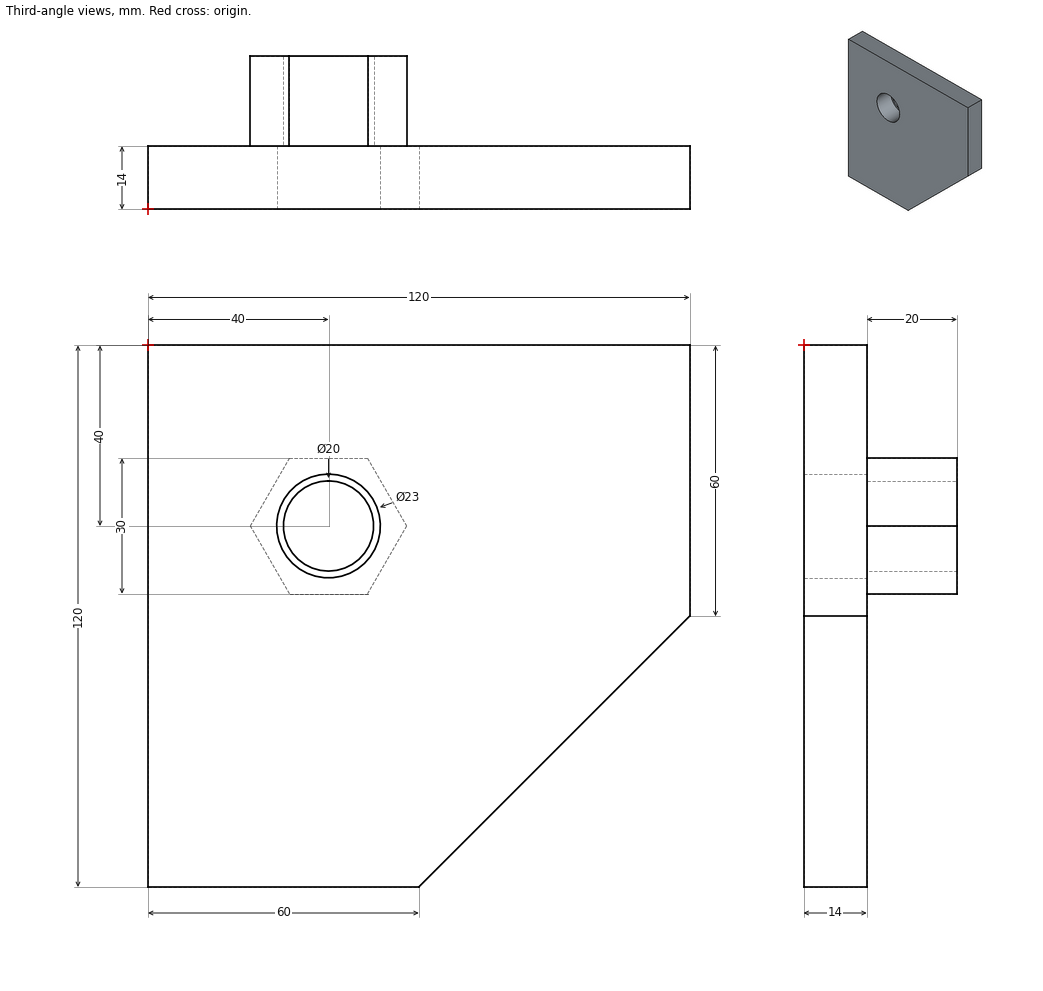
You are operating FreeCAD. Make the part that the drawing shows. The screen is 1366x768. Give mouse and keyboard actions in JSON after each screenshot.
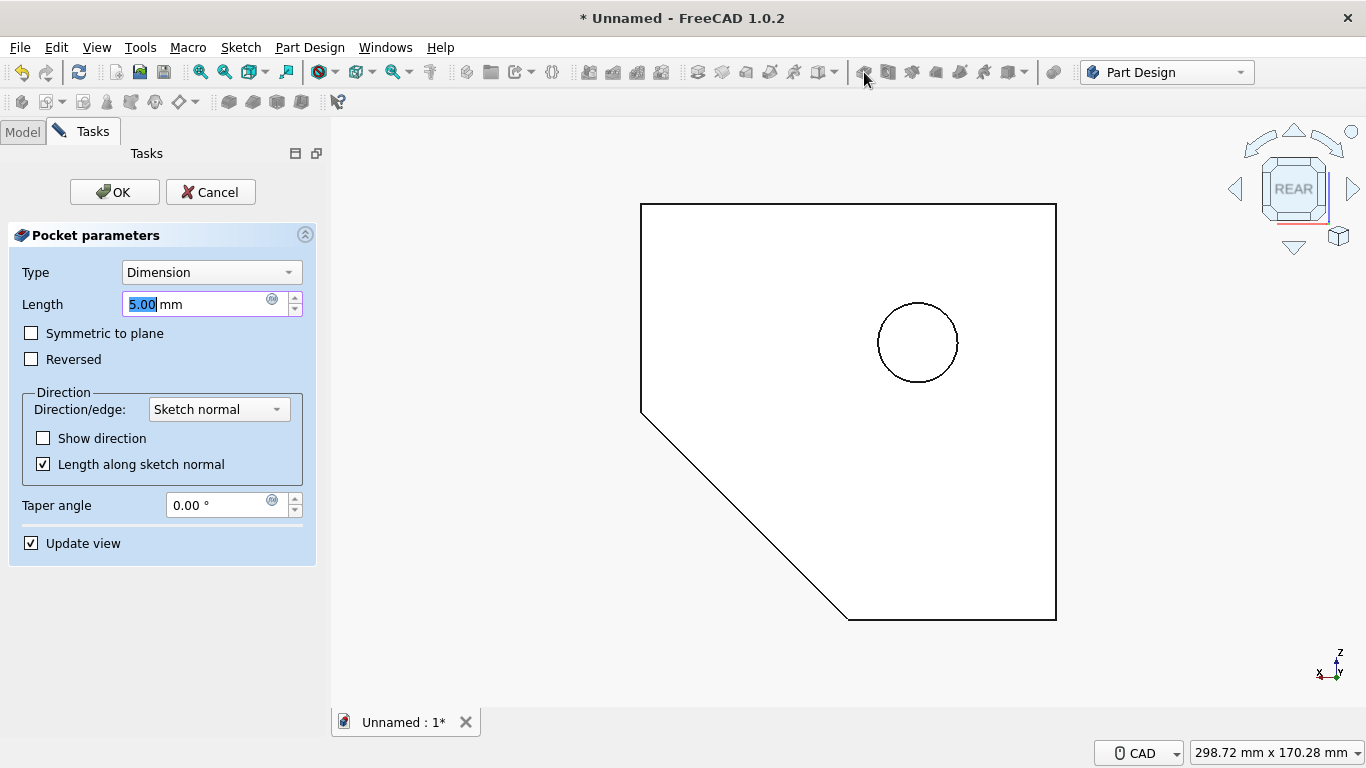
{"action": "type", "text": "14"}
{"action": "key", "text": "Tab"}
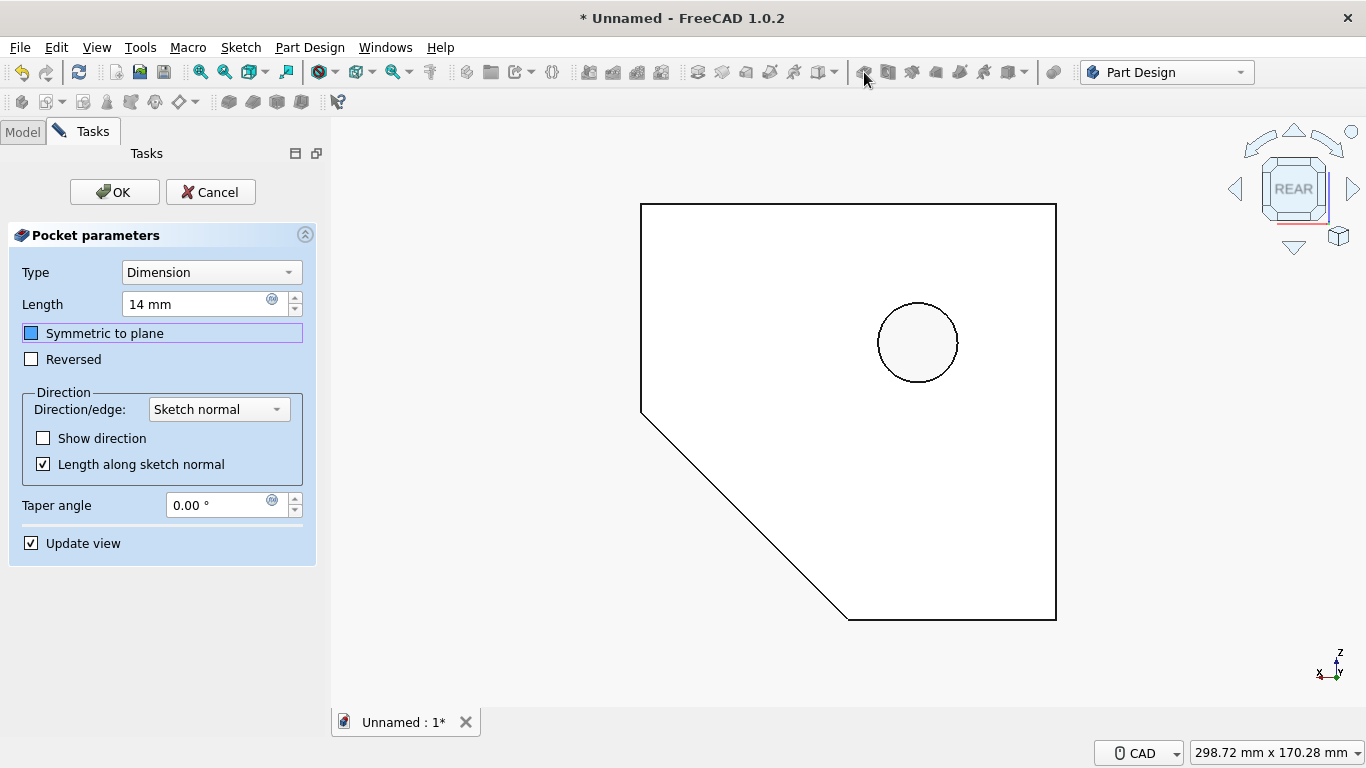
{"action": "left_click", "coordinate": [115, 192]}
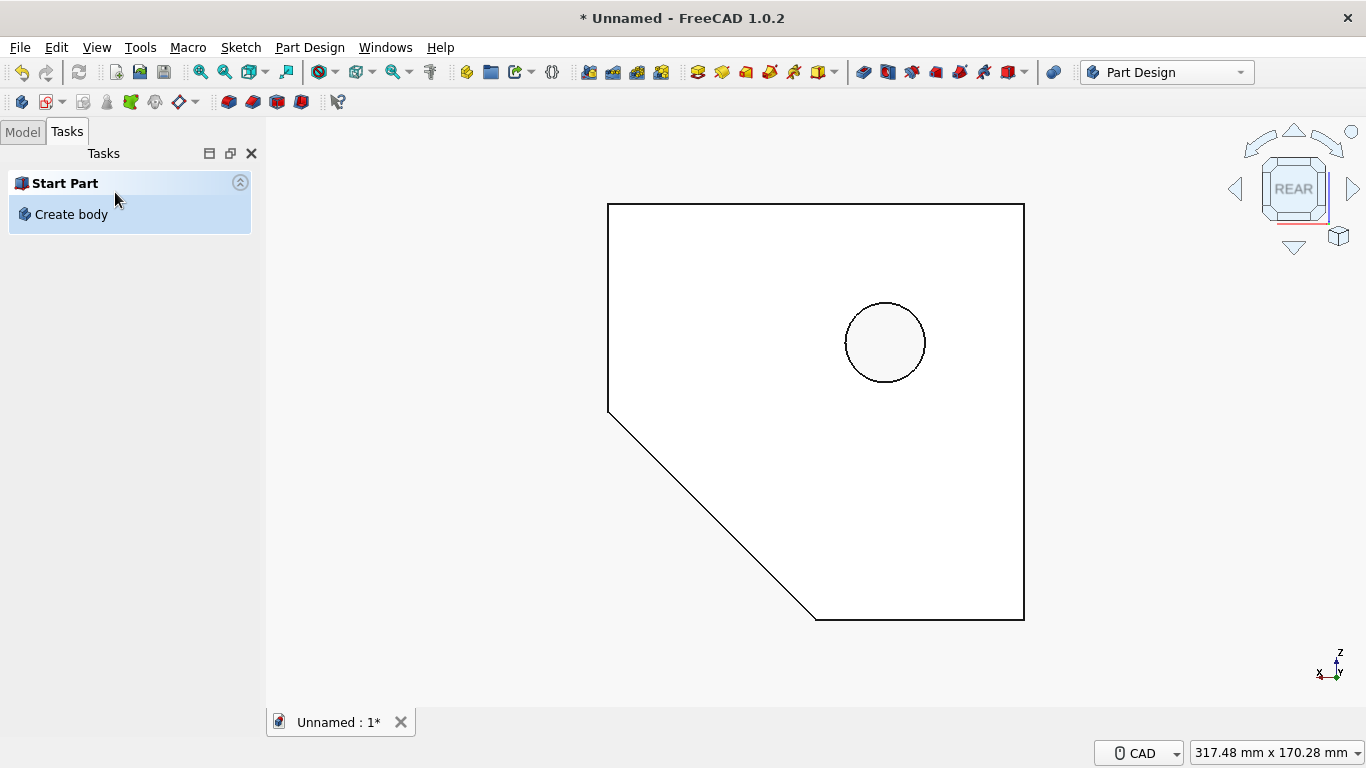
{"action": "left_click", "coordinate": [757, 411]}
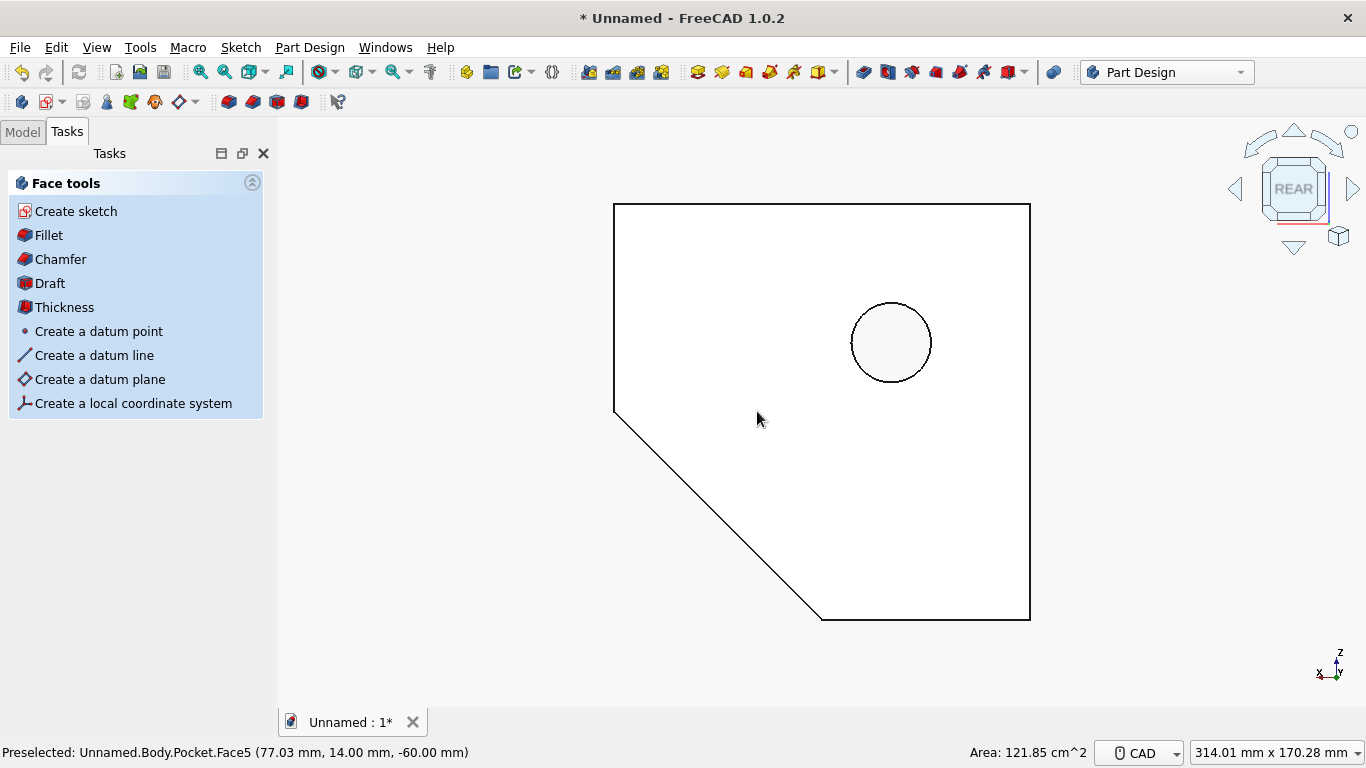
{"action": "left_click", "coordinate": [46, 102]}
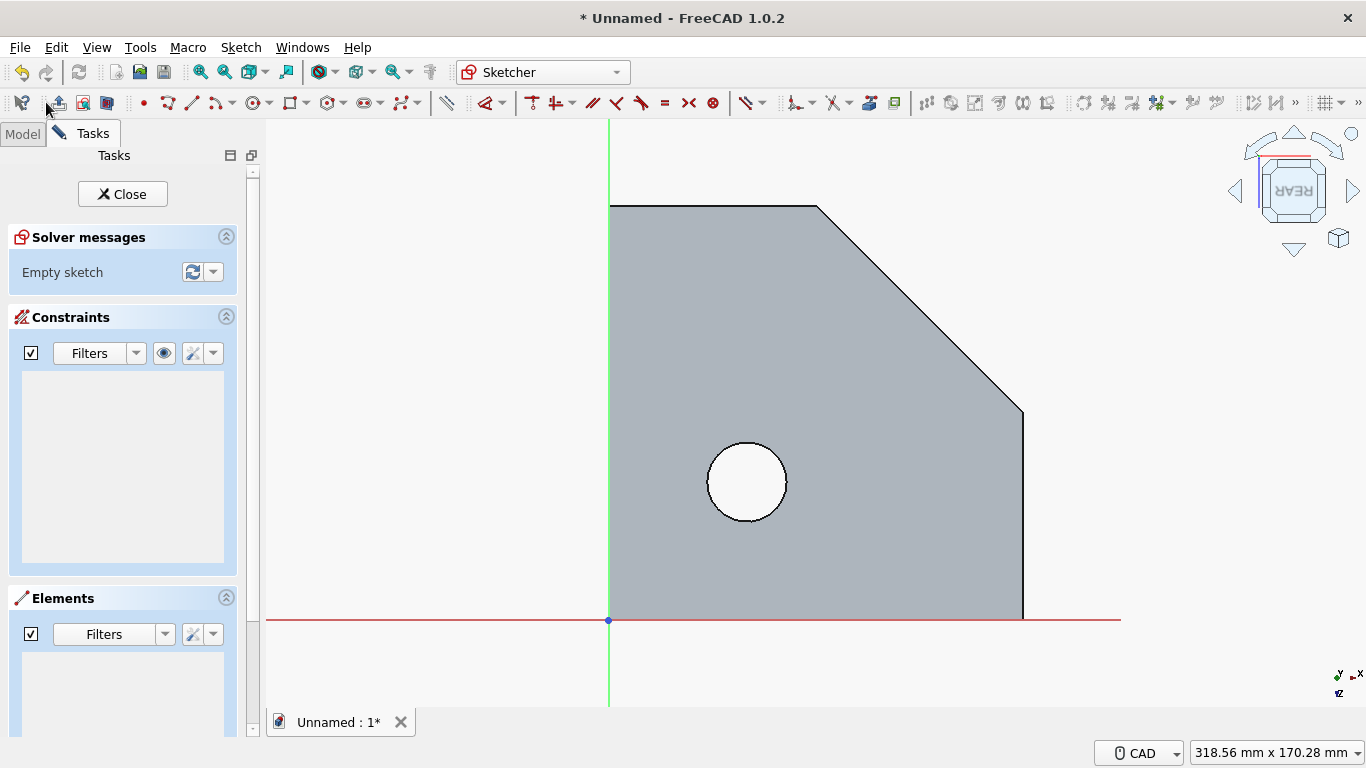
{"action": "scroll", "coordinate": [659, 662], "scroll_direction": "up", "scroll_amount": 3}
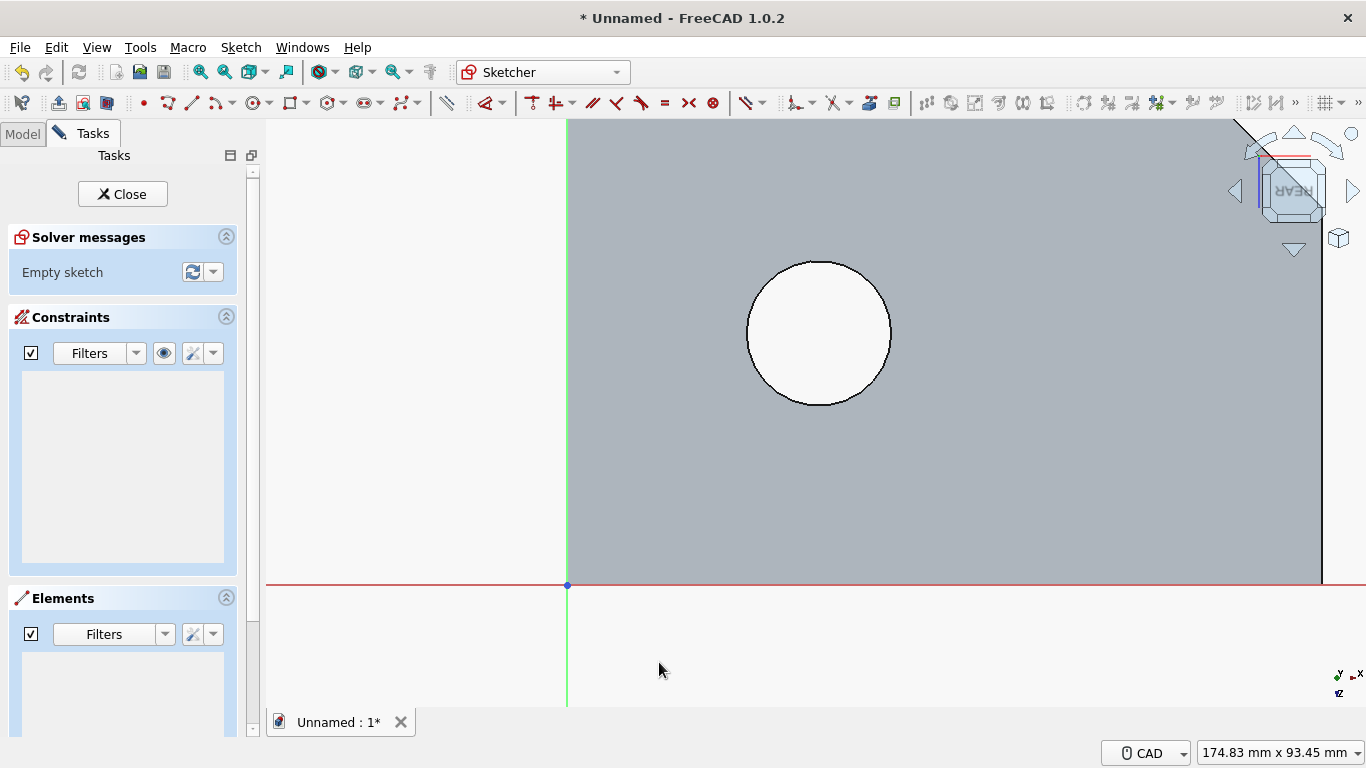
{"action": "left_click", "coordinate": [328, 104]}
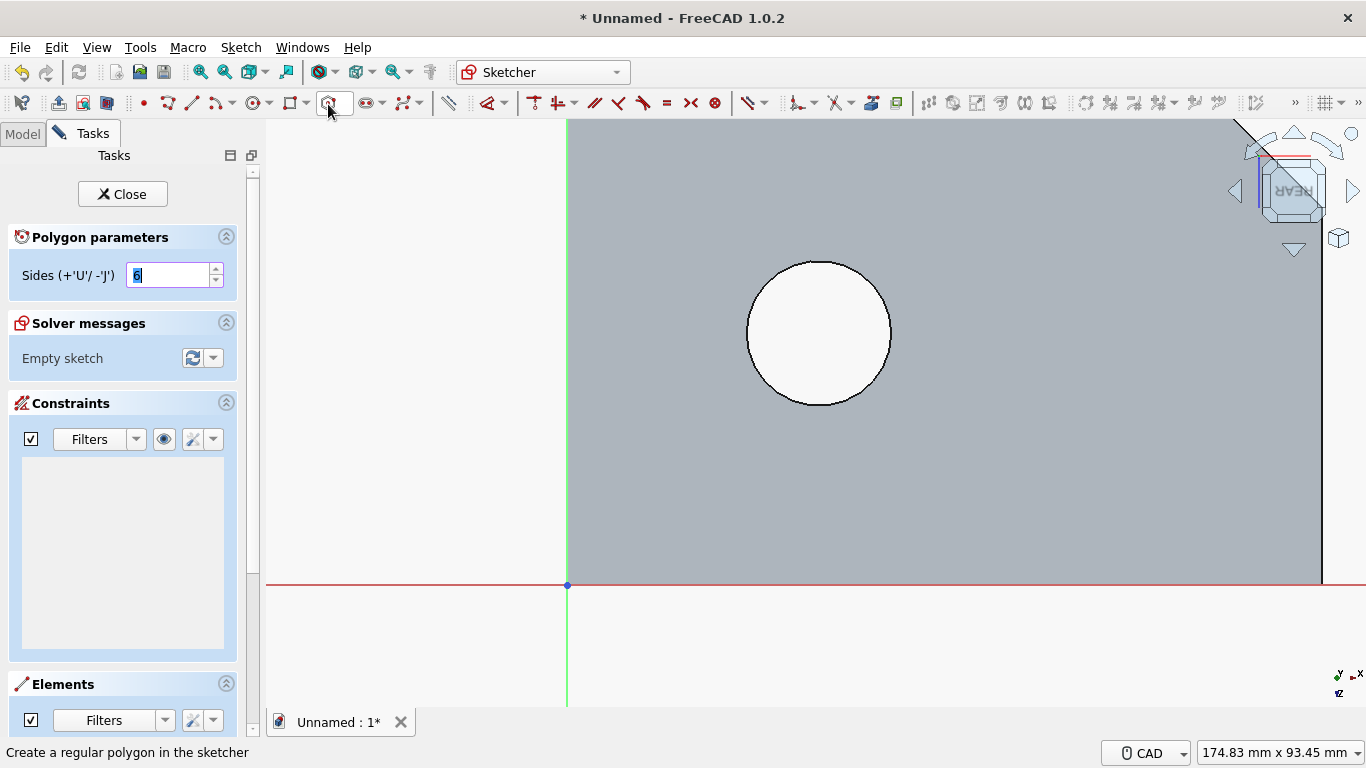
{"action": "left_click", "coordinate": [819, 333]}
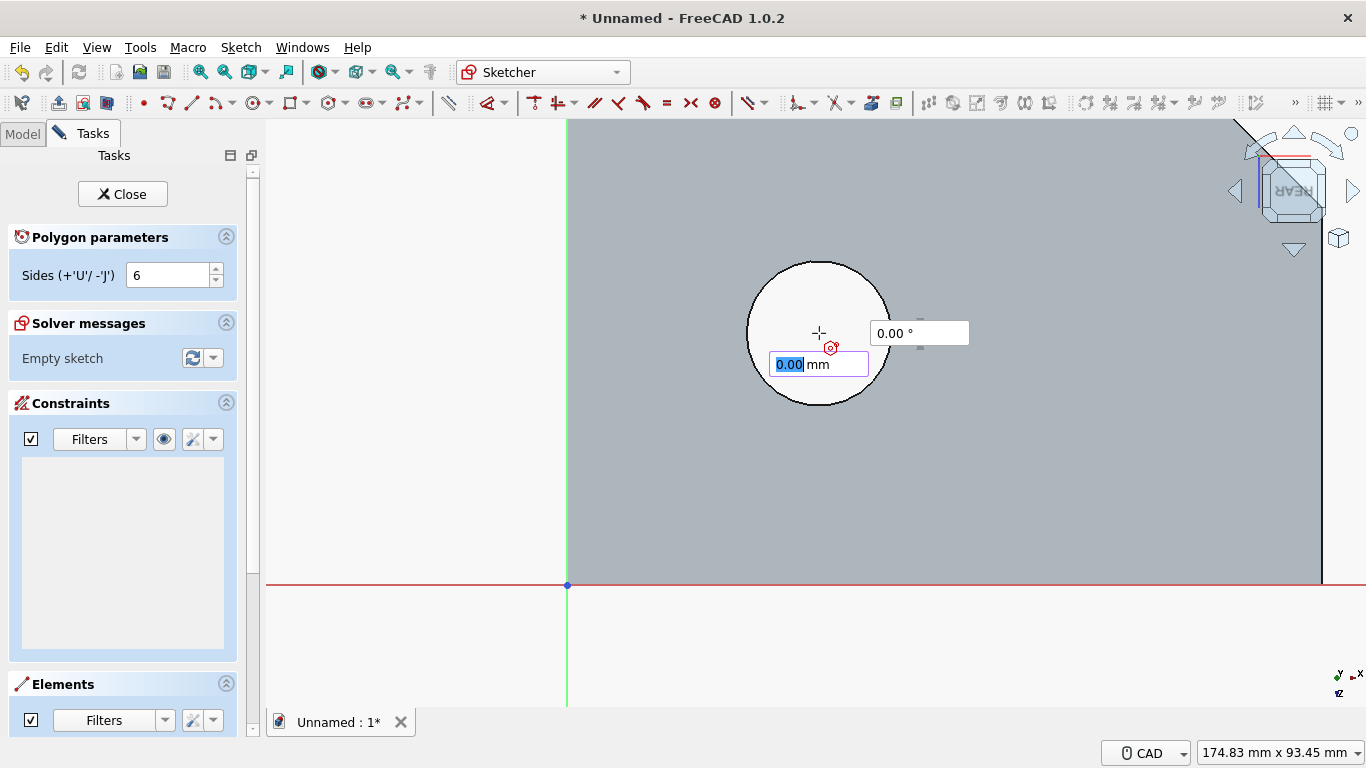
{"action": "left_click", "coordinate": [928, 333]}
{"action": "right_click", "coordinate": [928, 333]}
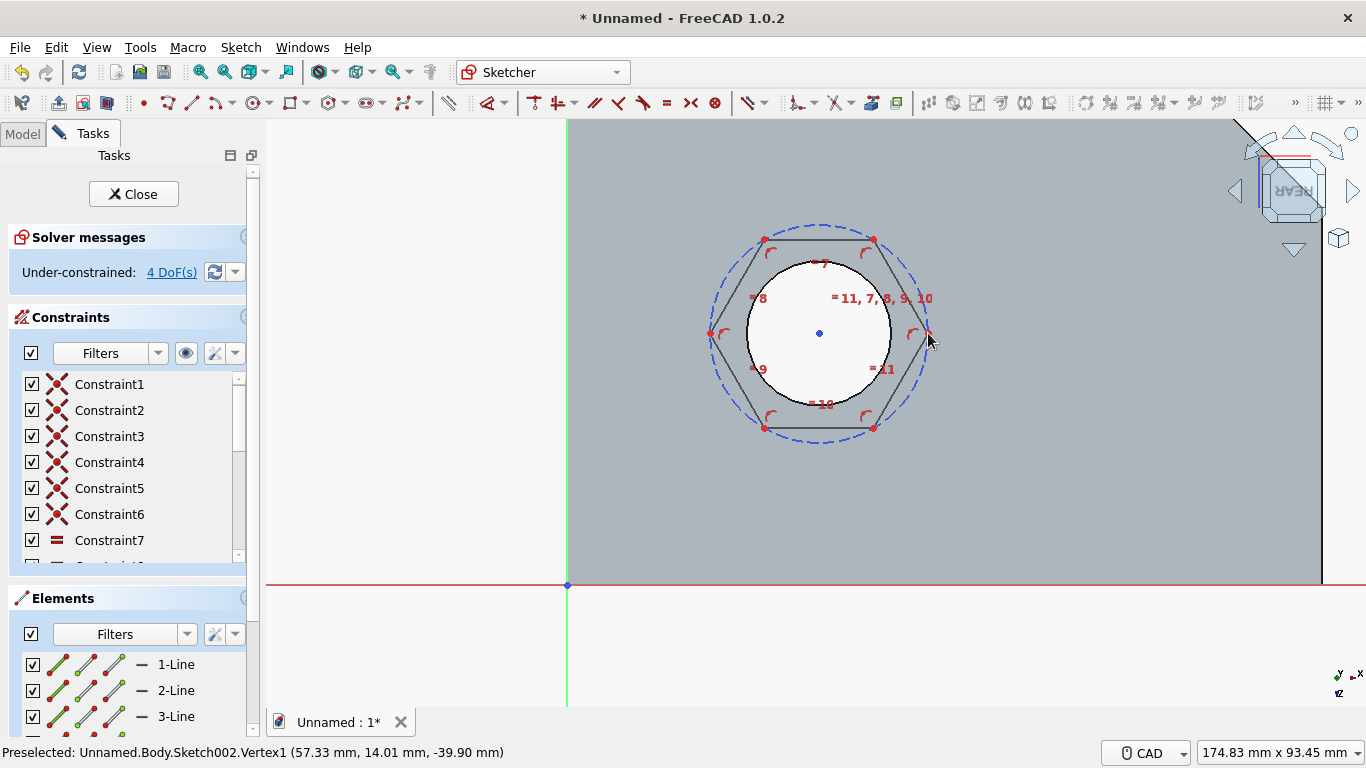
{"action": "left_click", "coordinate": [254, 104]}